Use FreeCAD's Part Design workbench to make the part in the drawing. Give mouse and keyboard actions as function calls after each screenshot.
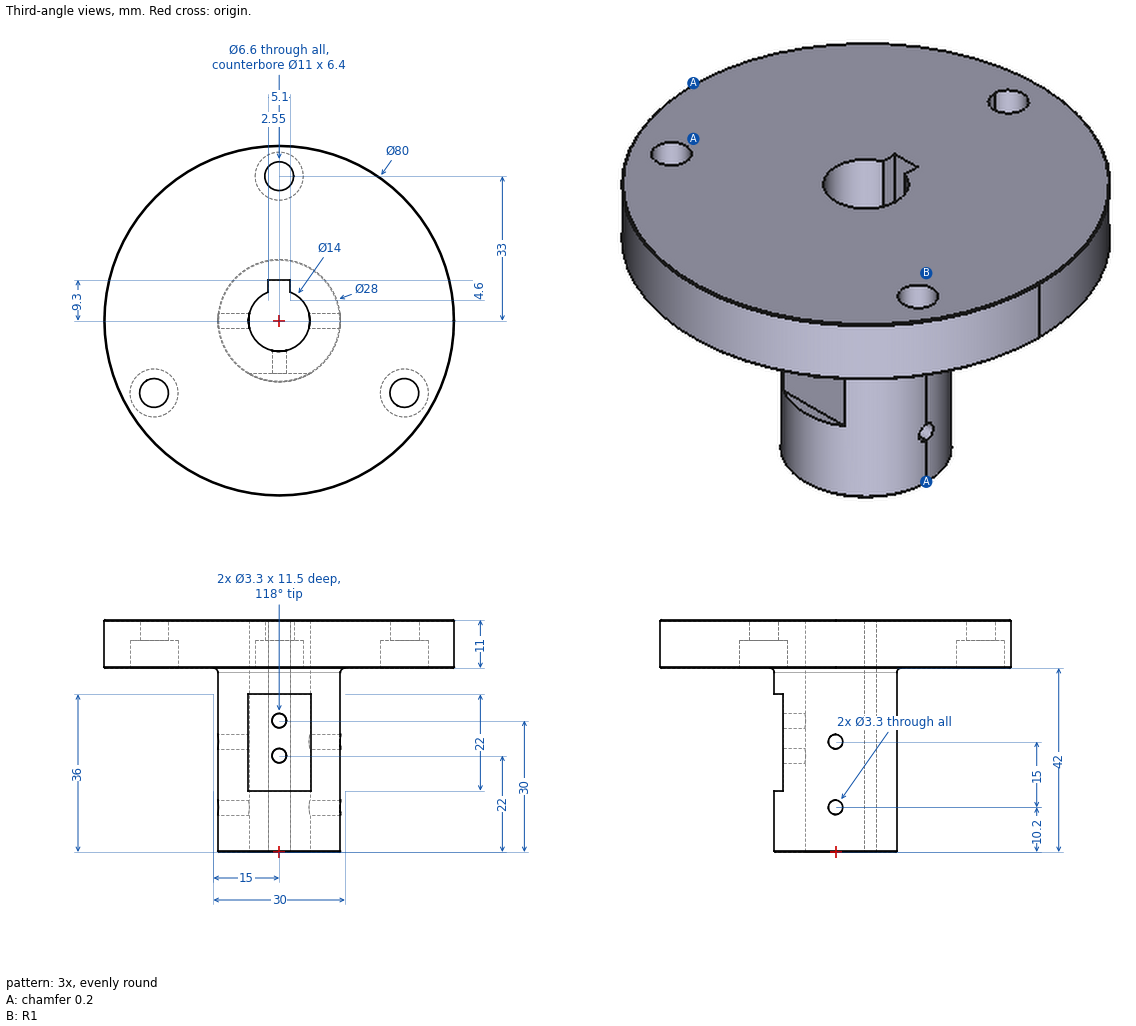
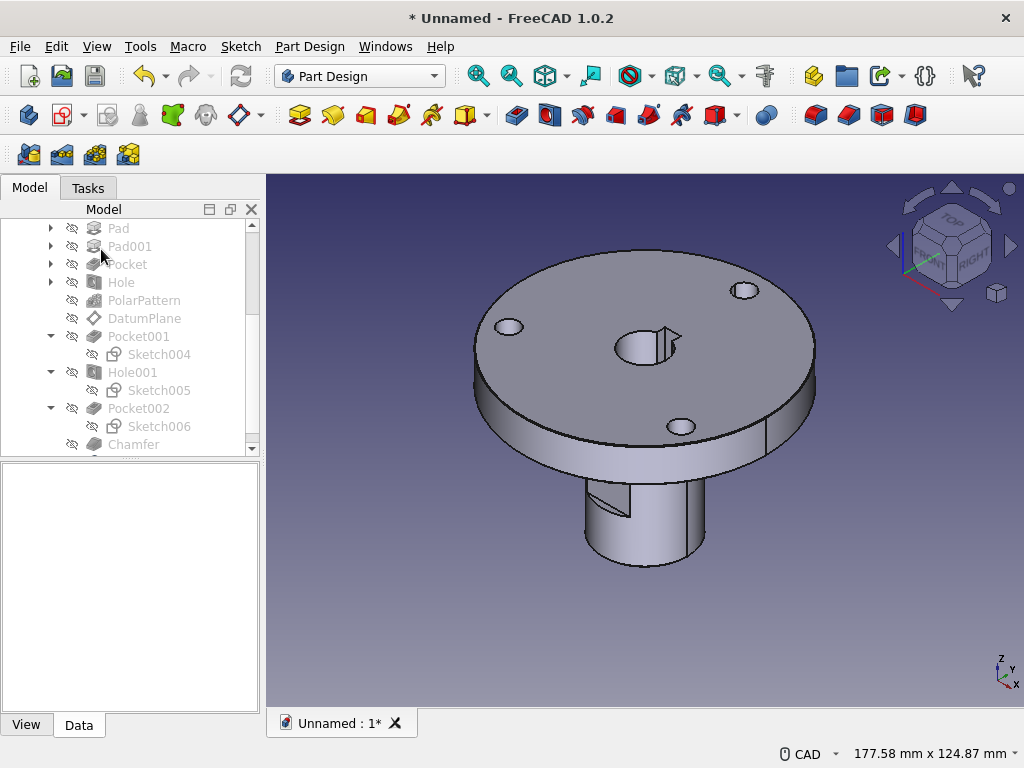
scroll(141, 332, down, 3)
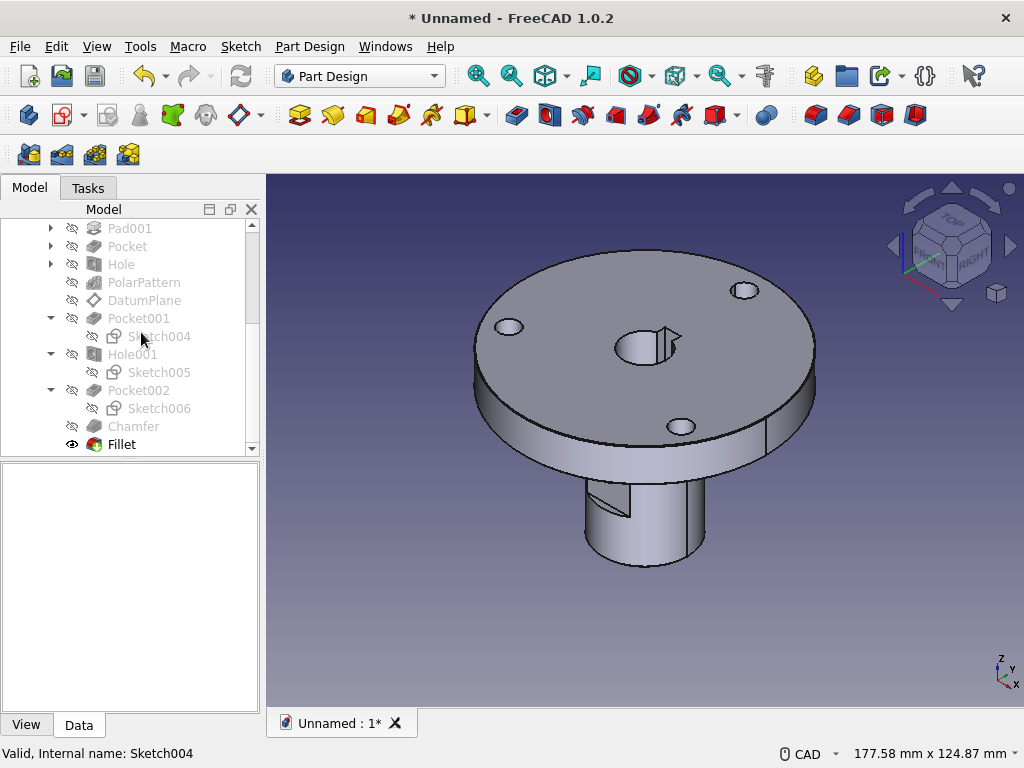
scroll(141, 332, up, 15)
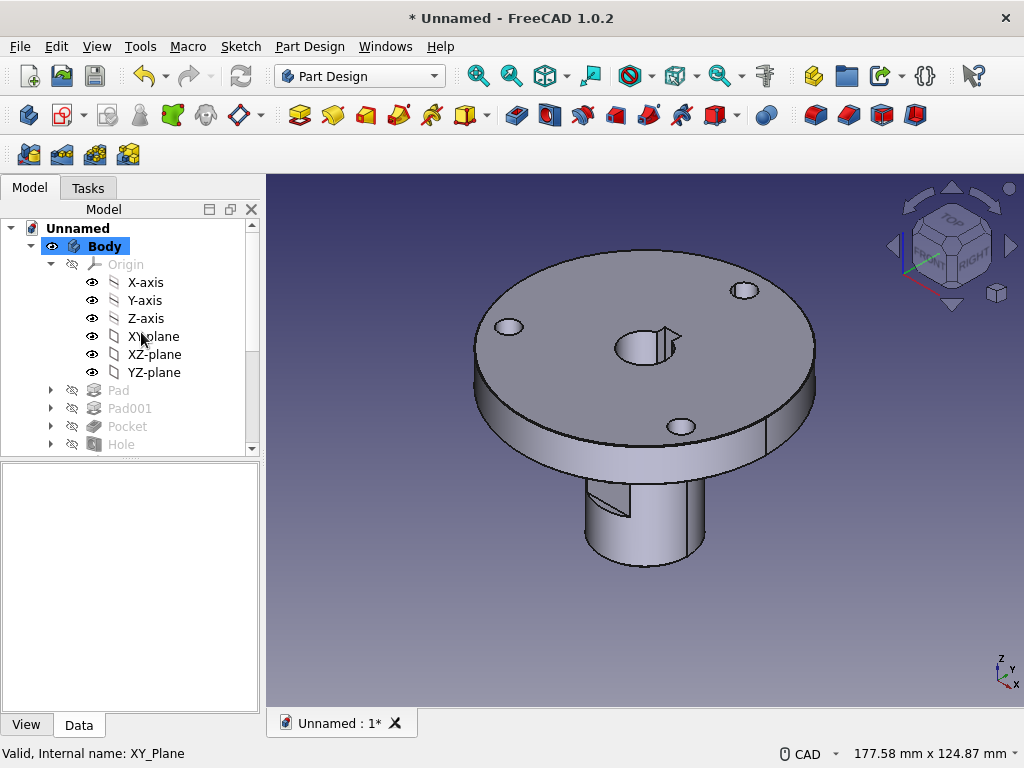
click(137, 372)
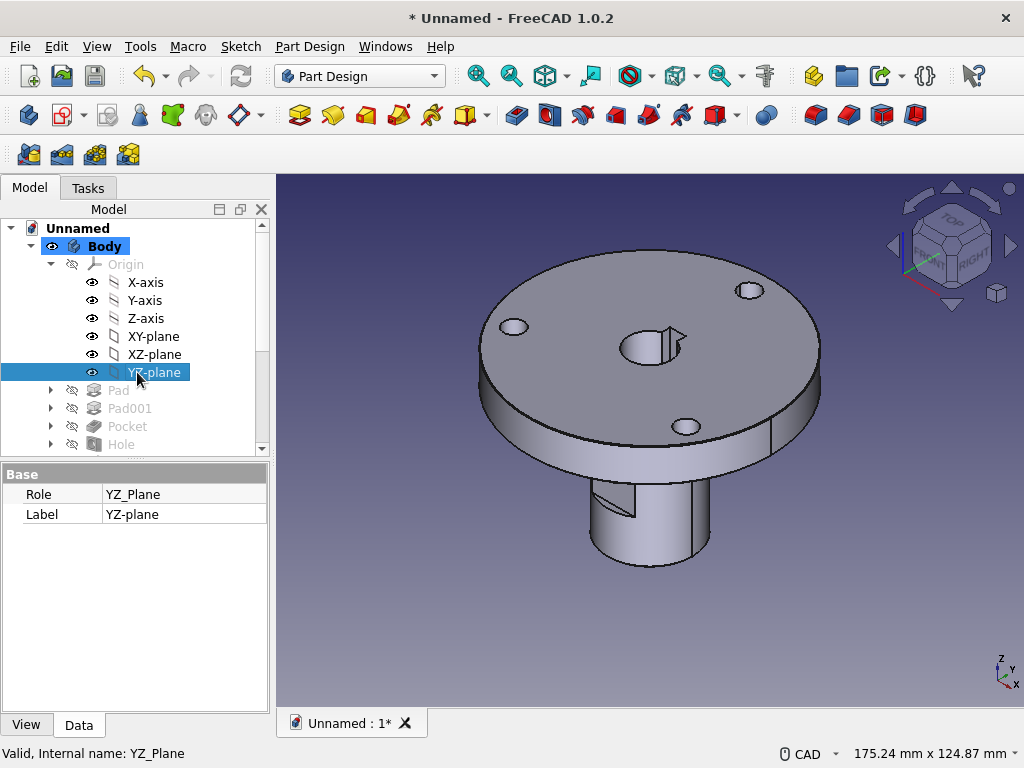
click(238, 116)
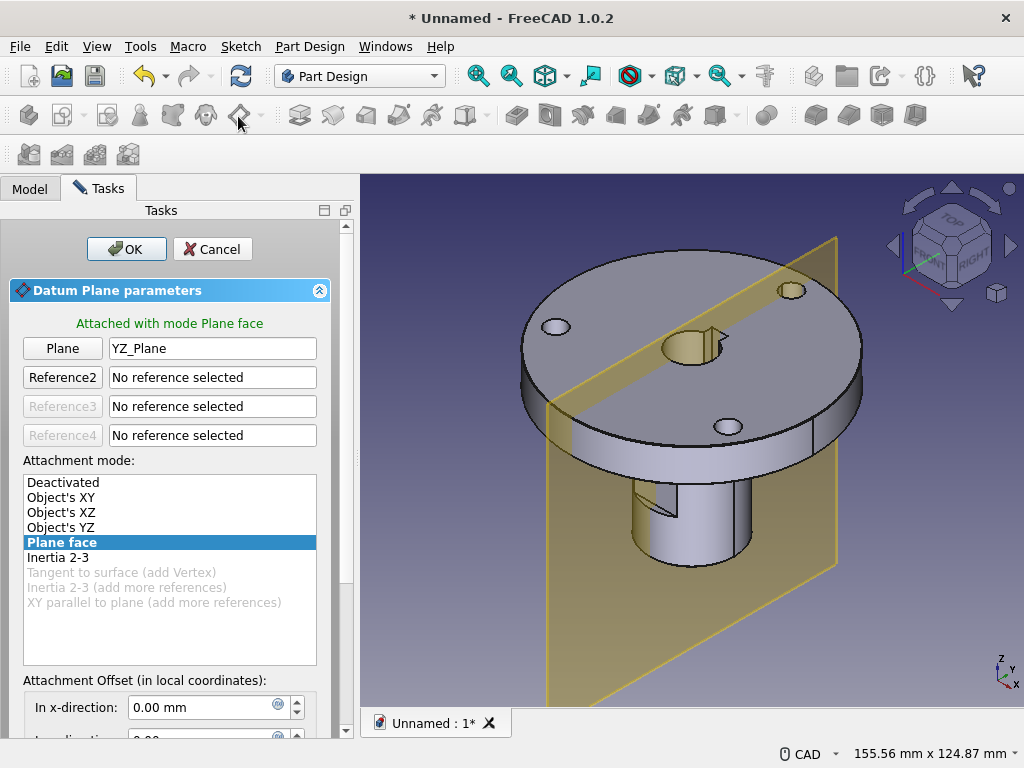
scroll(346, 479, down, 2)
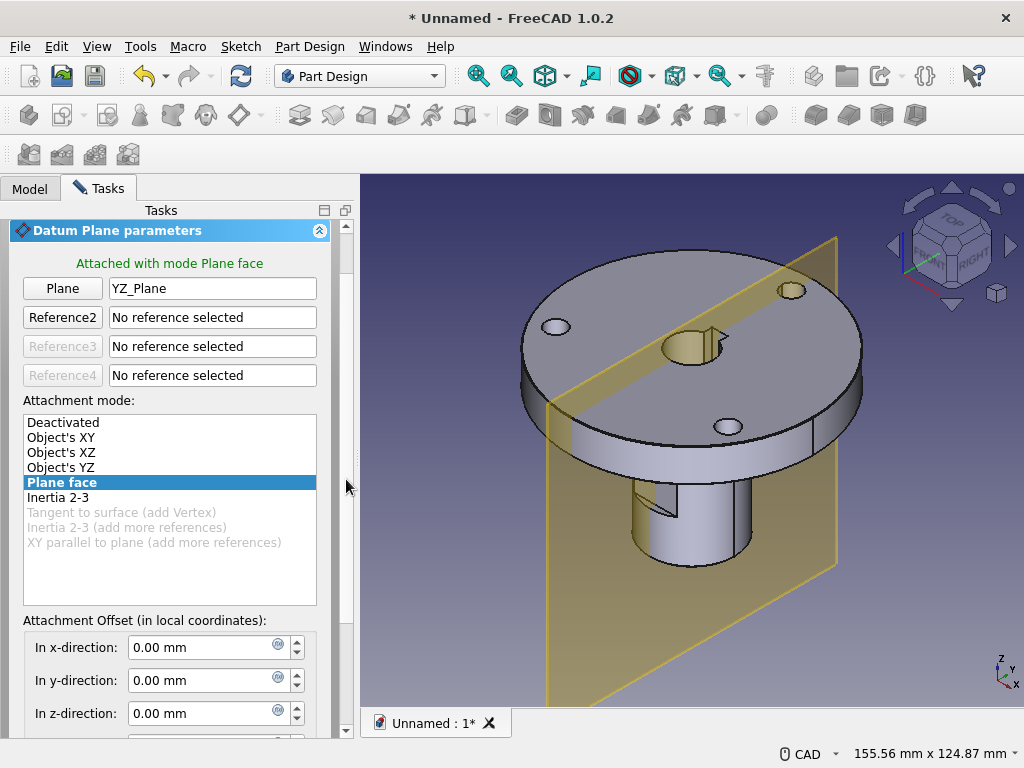
triple_click(210, 654)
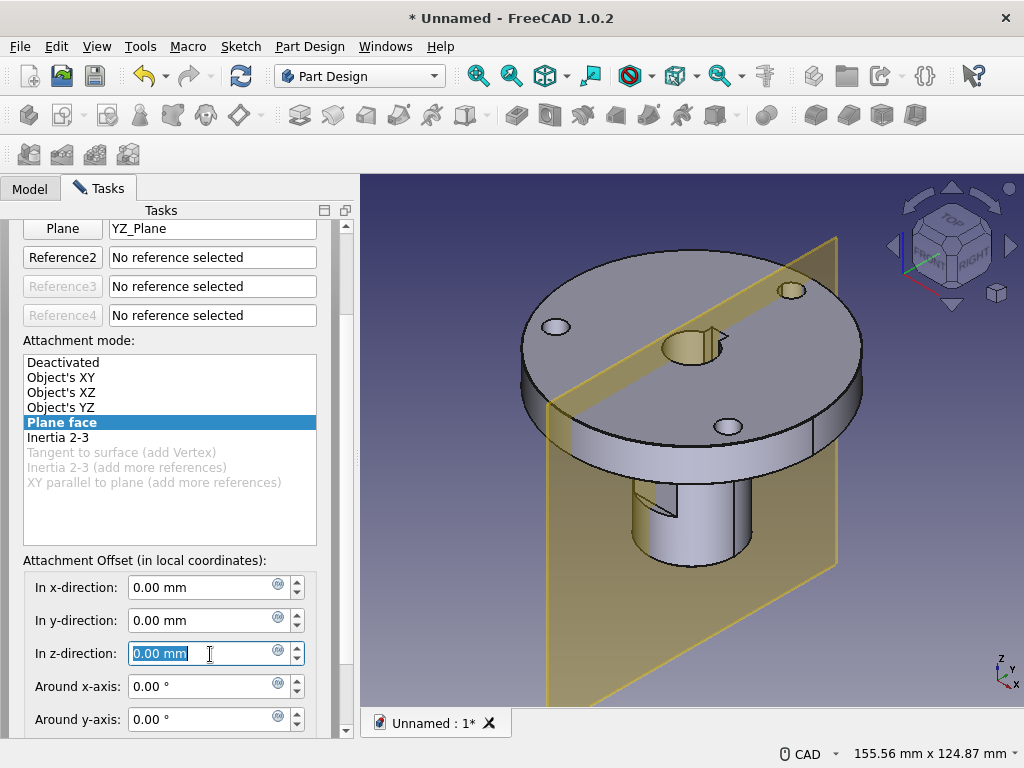
text(15)
key(Tab)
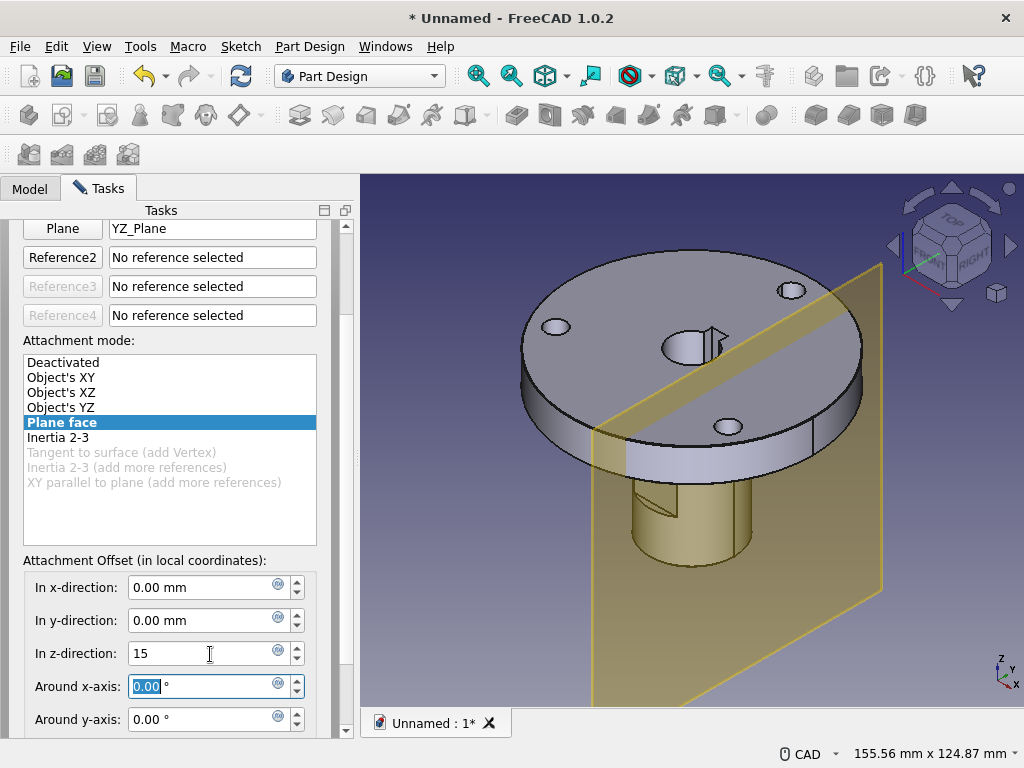
scroll(346, 479, up, 3)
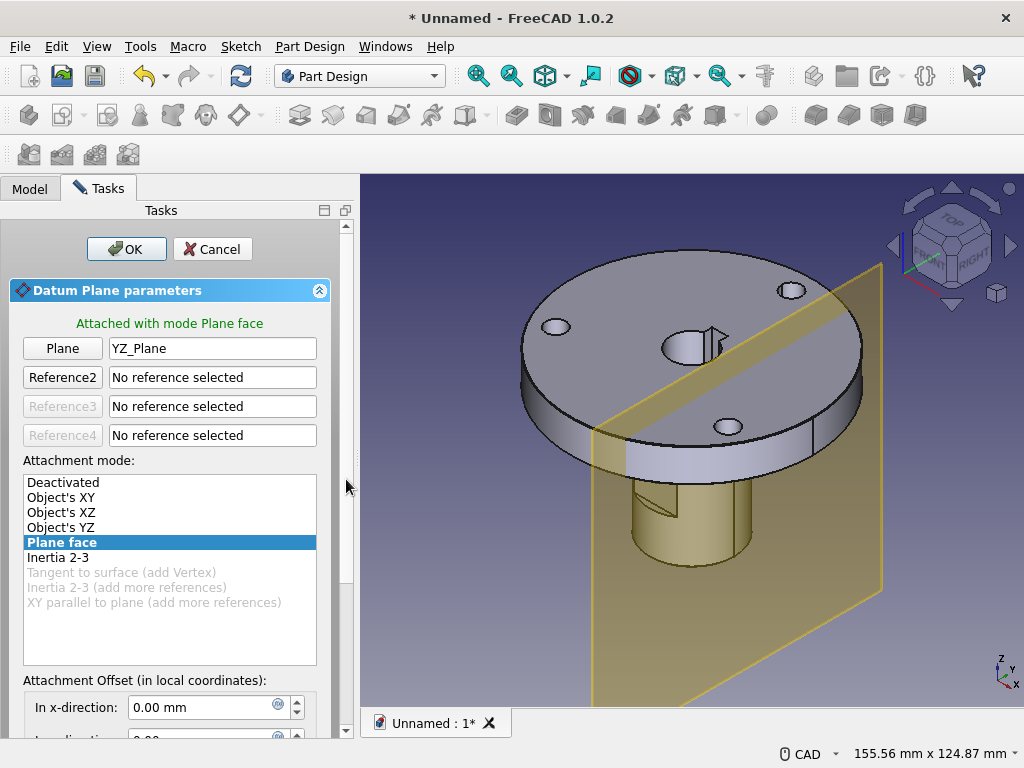
click(127, 249)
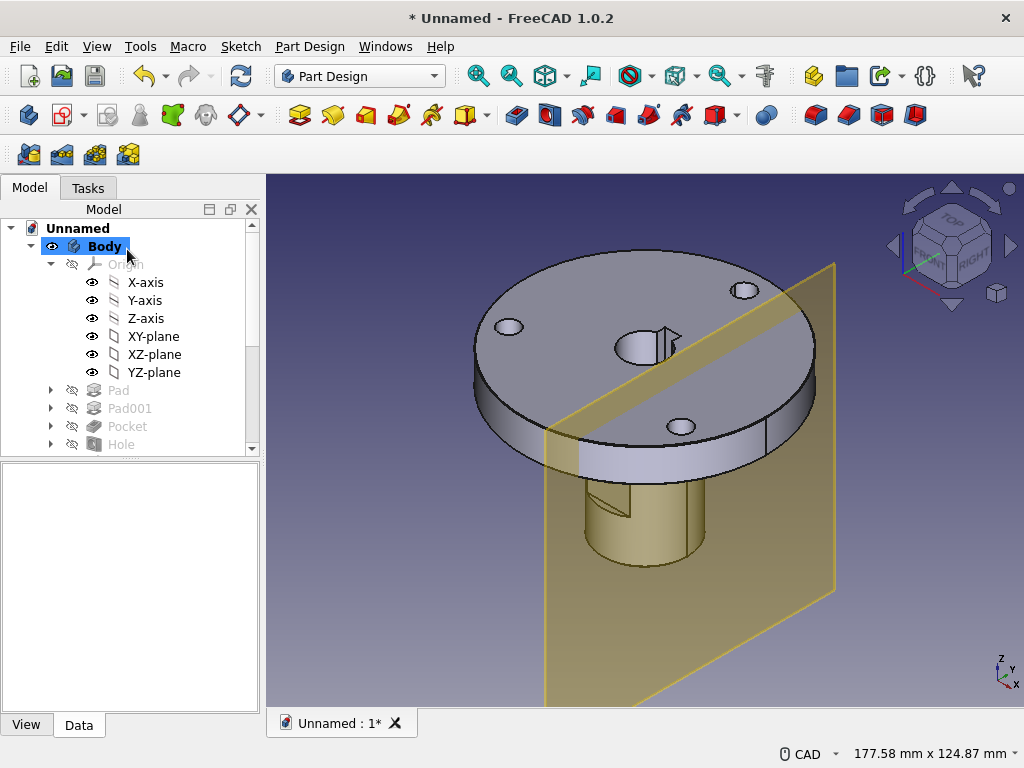
scroll(101, 332, down, 3)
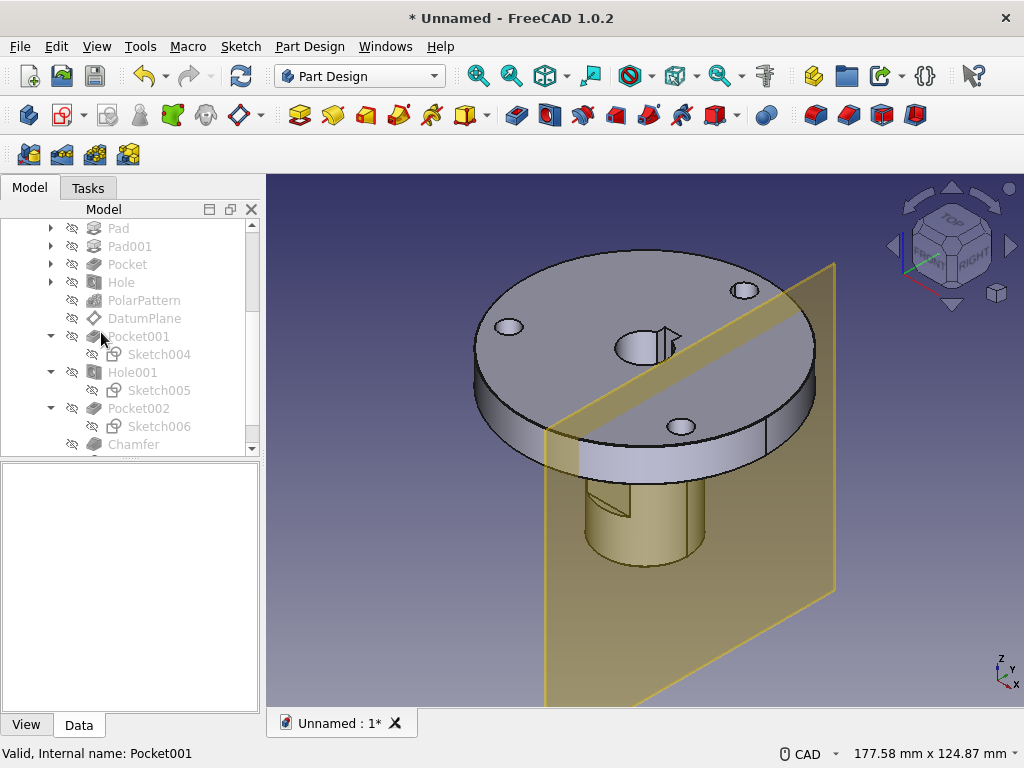
scroll(141, 332, up, 15)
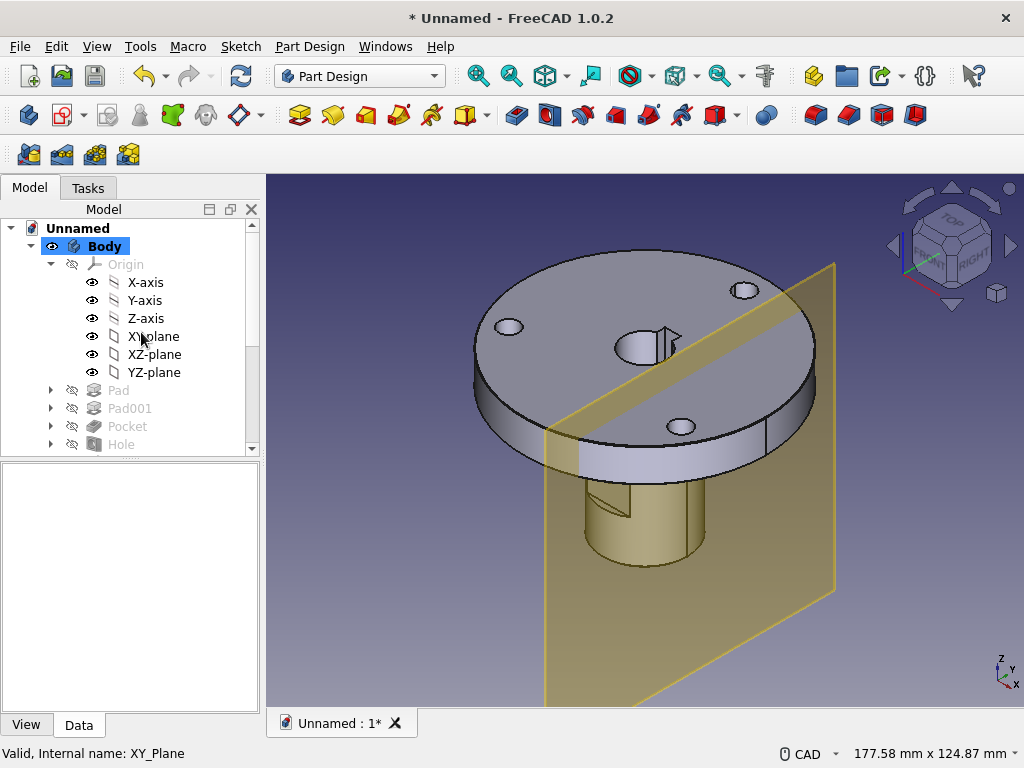
scroll(101, 332, down, 6)